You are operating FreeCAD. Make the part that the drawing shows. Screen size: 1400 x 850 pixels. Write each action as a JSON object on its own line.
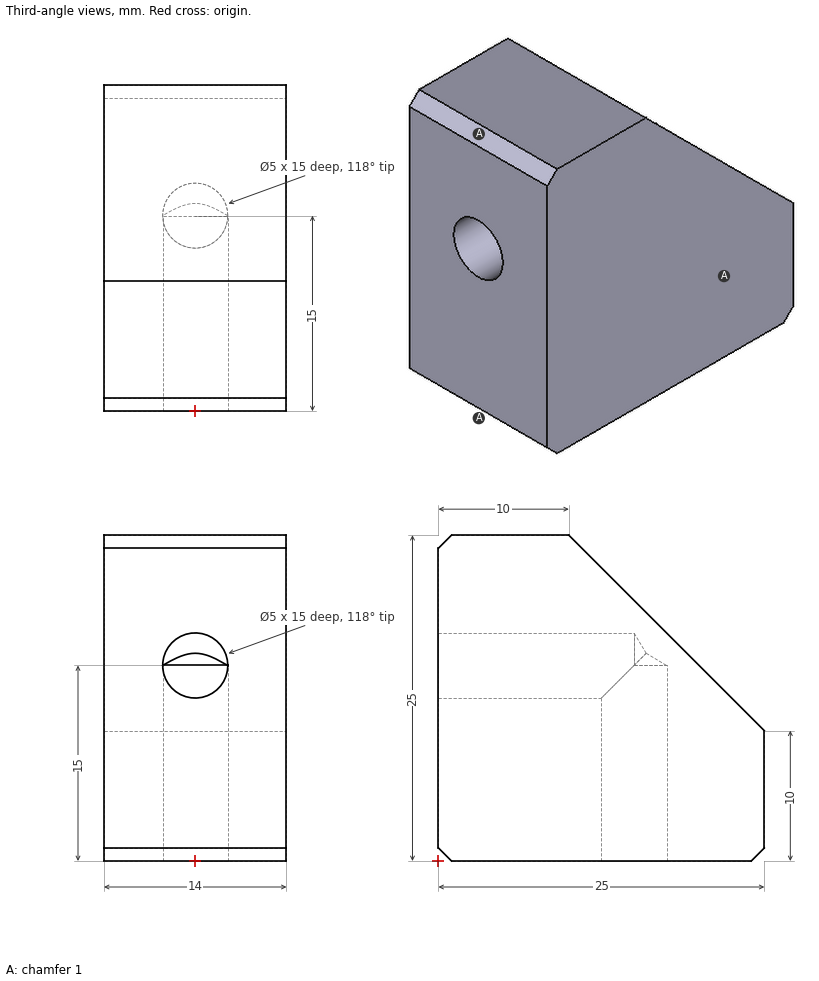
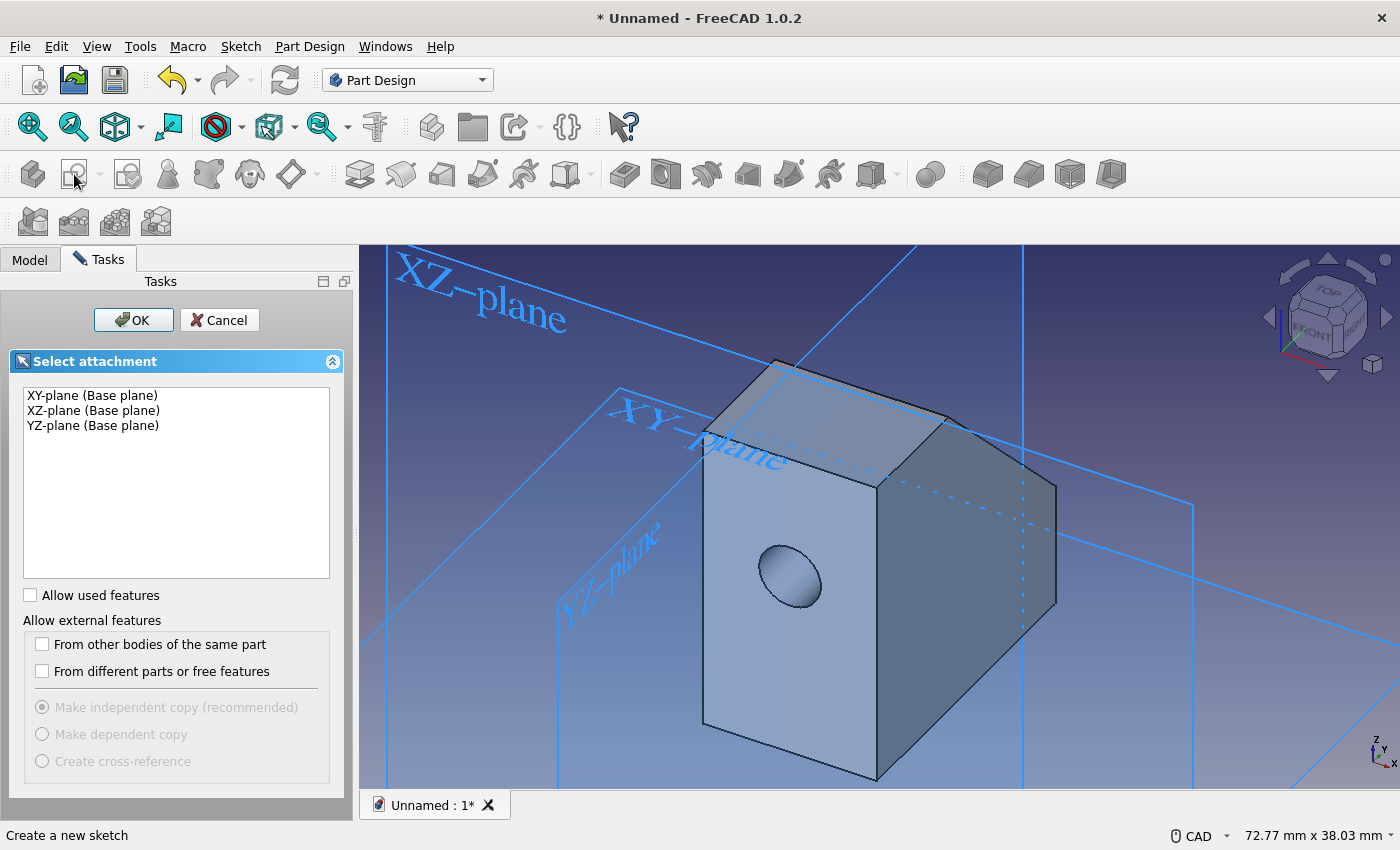
{"action": "left_click", "coordinate": [84, 396]}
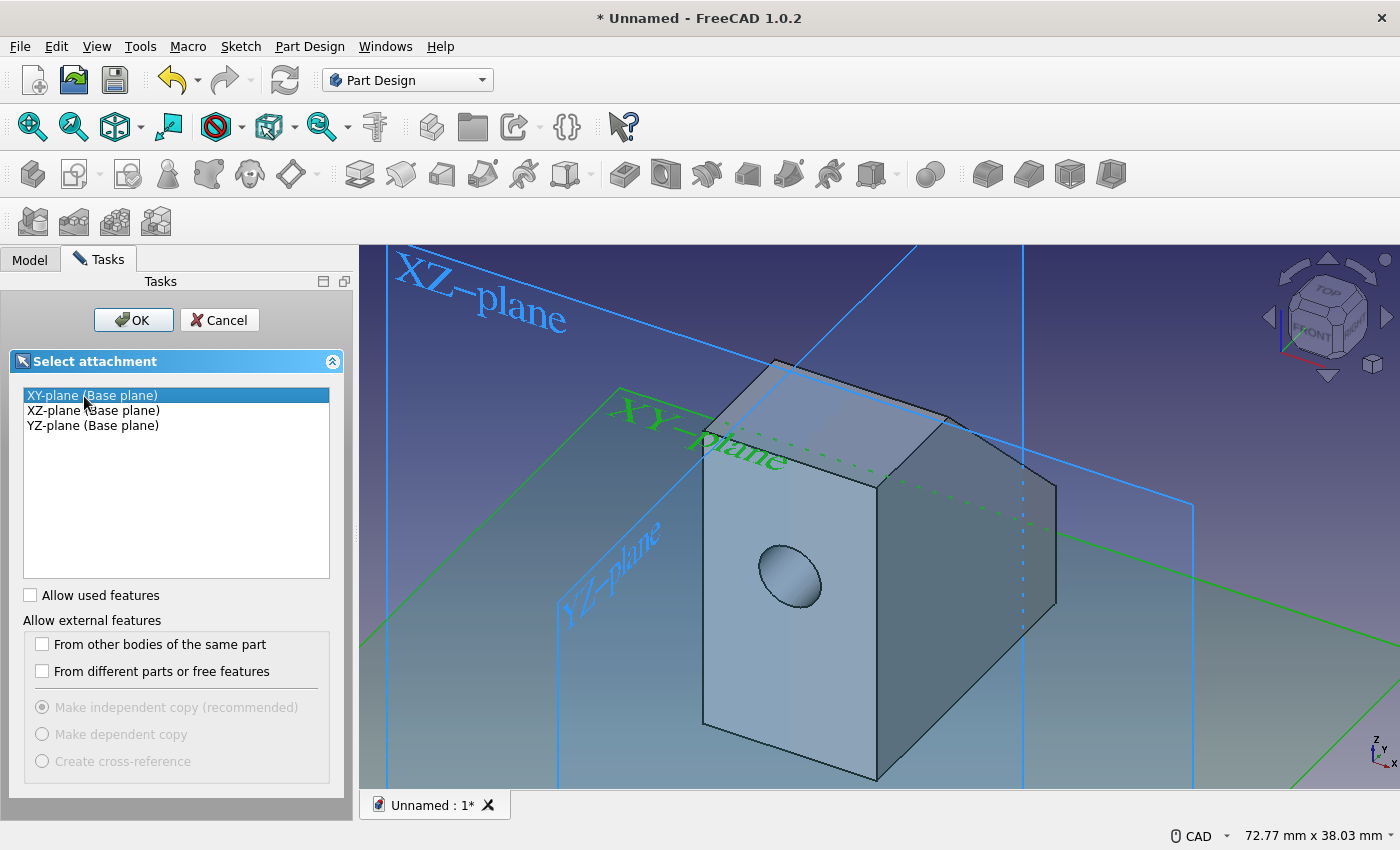
{"action": "left_click", "coordinate": [134, 320]}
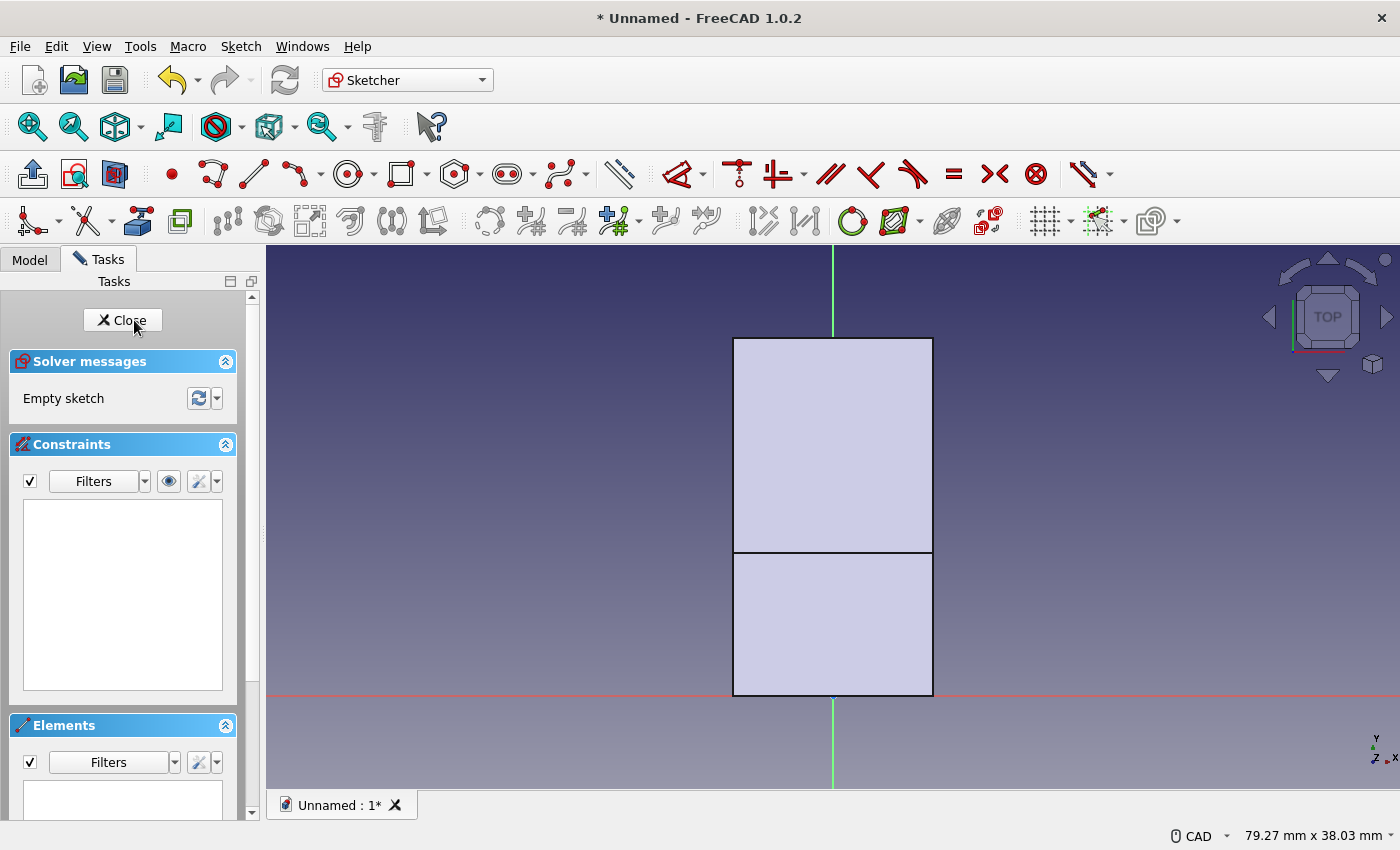
{"action": "left_click", "coordinate": [115, 174]}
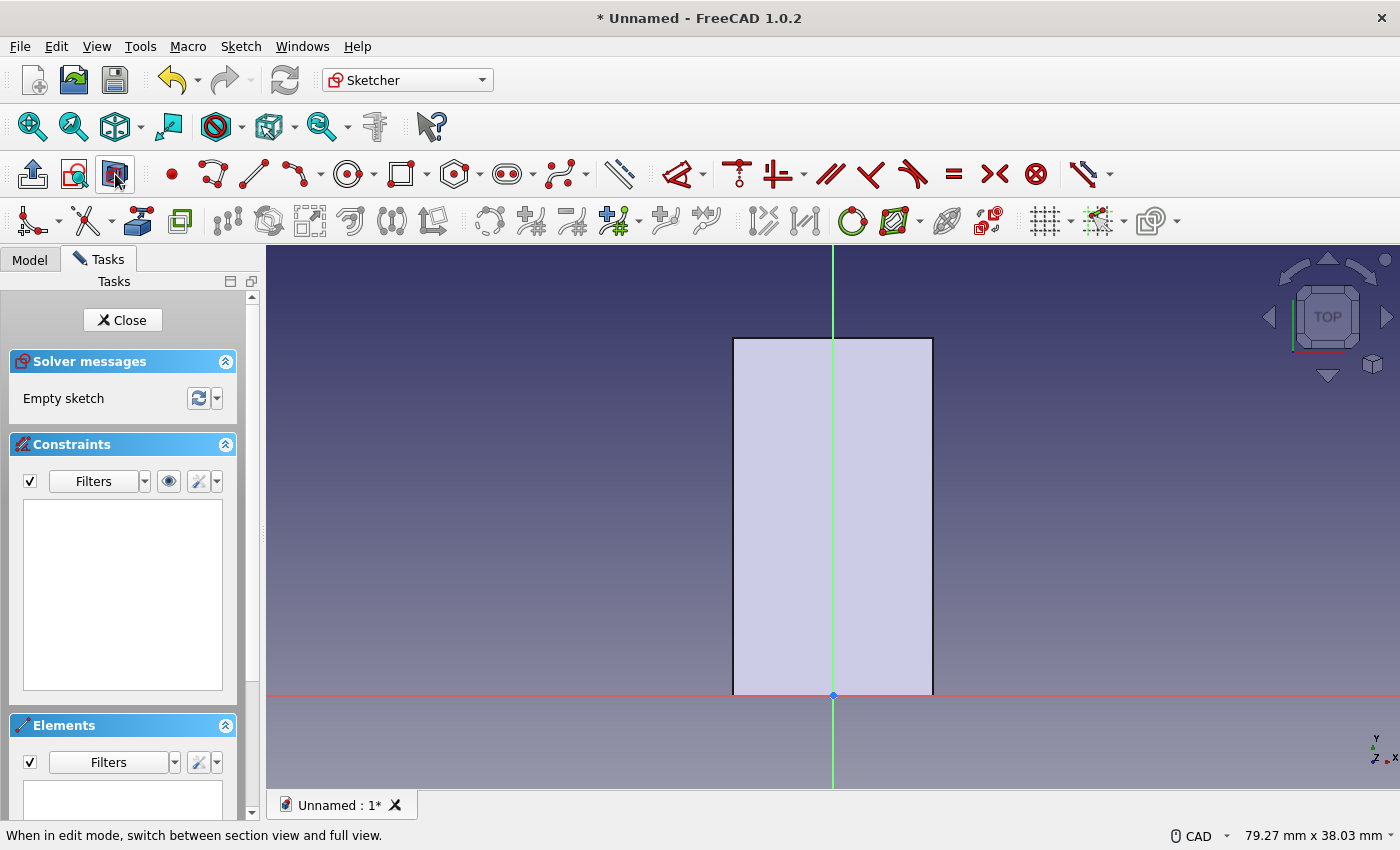
{"action": "scroll", "coordinate": [850, 472], "scroll_direction": "up", "scroll_amount": 8}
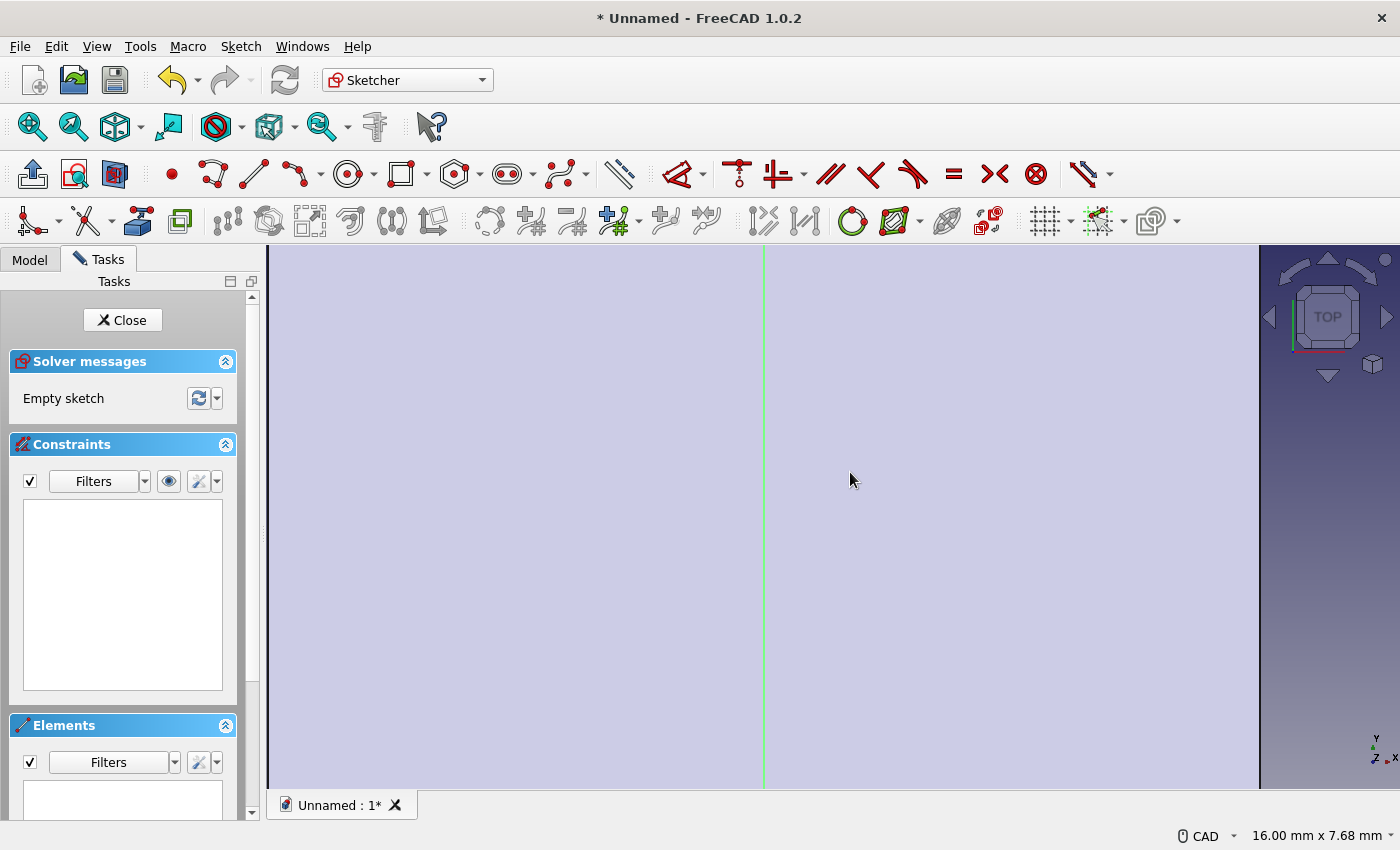
{"action": "left_click", "coordinate": [348, 174]}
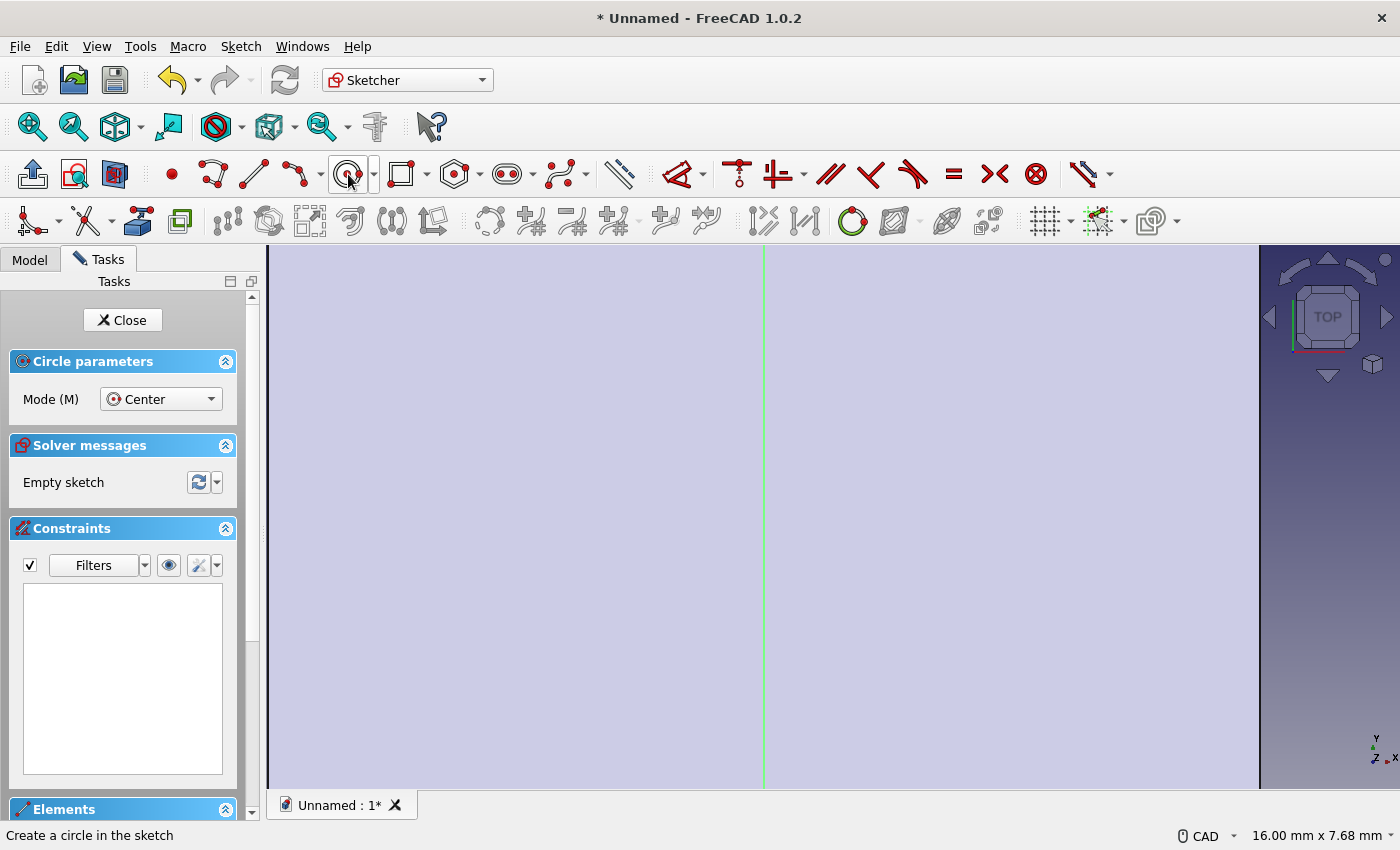
{"action": "left_click", "coordinate": [764, 516]}
{"action": "left_click", "coordinate": [889, 391]}
{"action": "key", "text": "Escape"}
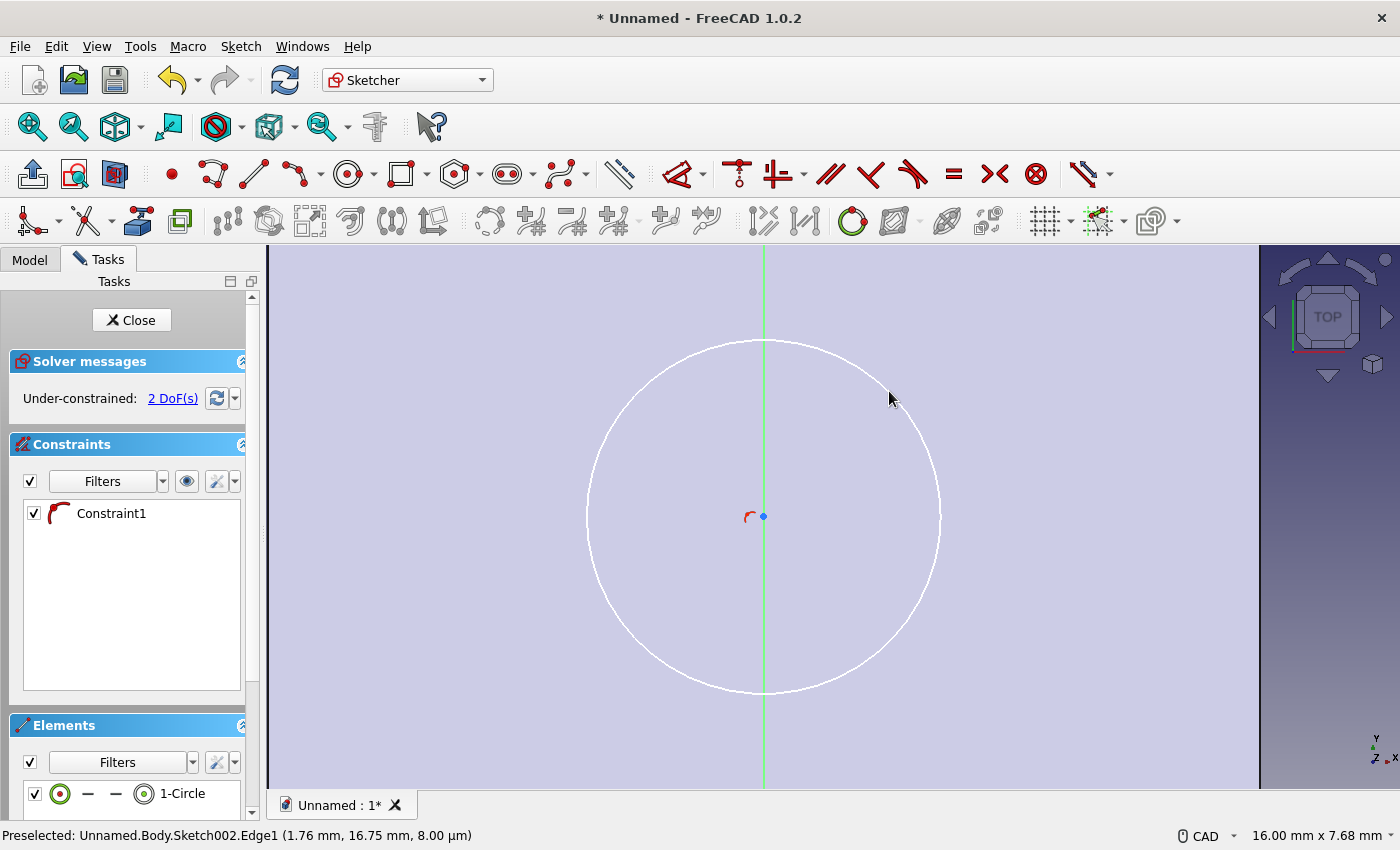
{"action": "left_click", "coordinate": [676, 174]}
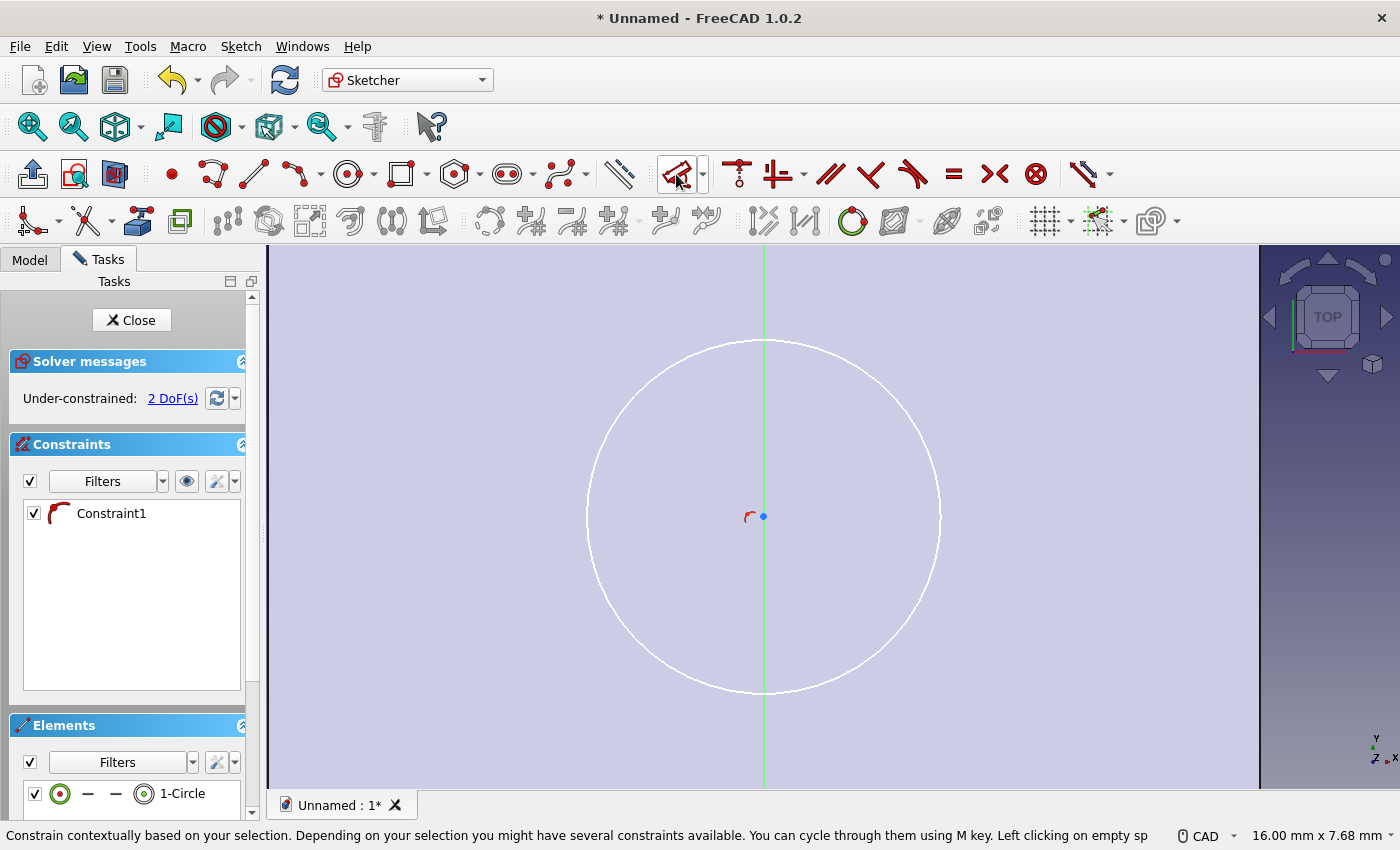
{"action": "left_click", "coordinate": [888, 391]}
{"action": "left_click", "coordinate": [910, 368]}